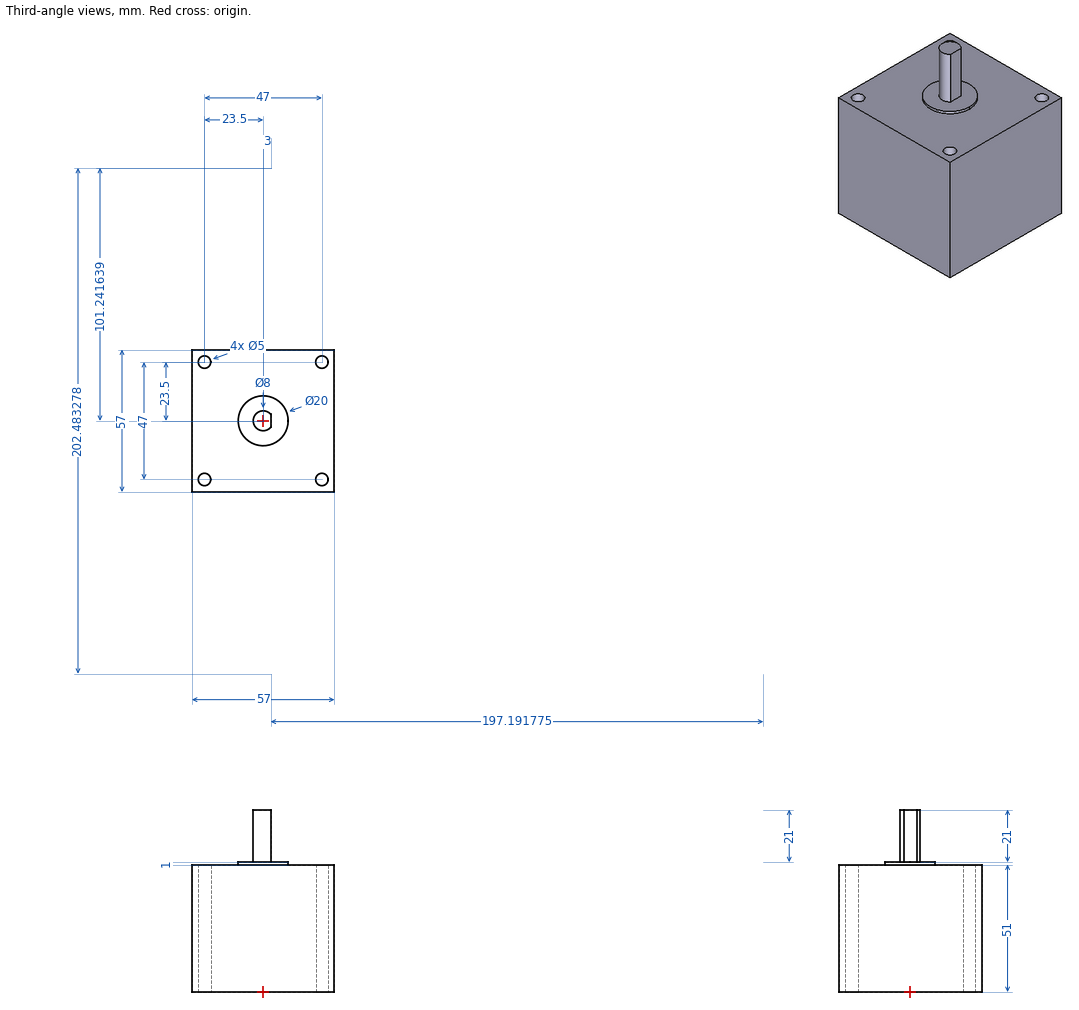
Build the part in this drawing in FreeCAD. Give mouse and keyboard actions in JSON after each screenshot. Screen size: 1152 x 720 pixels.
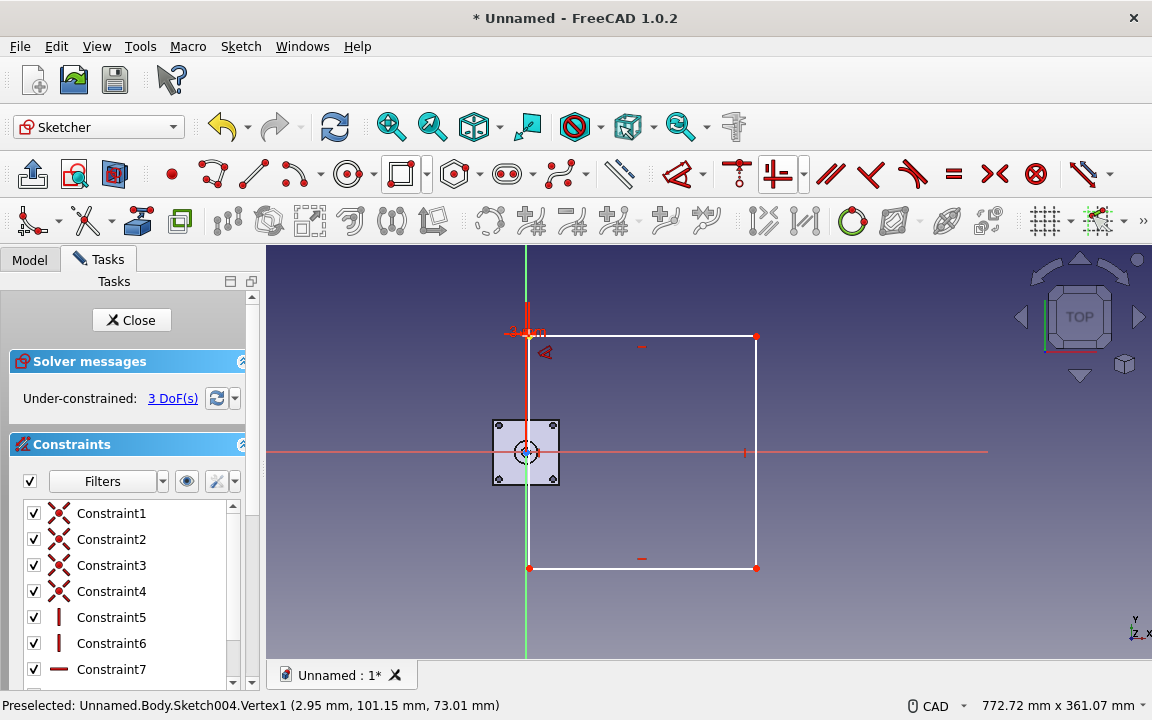
{"action": "scroll", "coordinate": [529, 406], "scroll_direction": "up", "scroll_amount": 7}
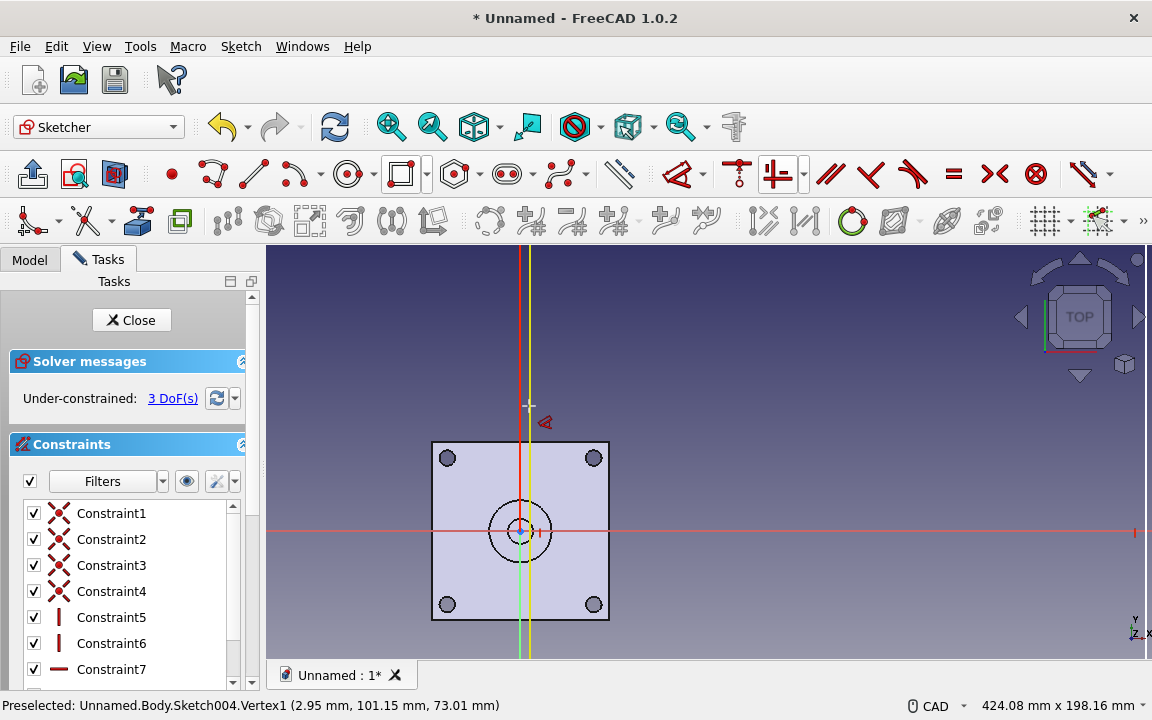
{"action": "left_click", "coordinate": [530, 405]}
{"action": "left_click", "coordinate": [496, 452]}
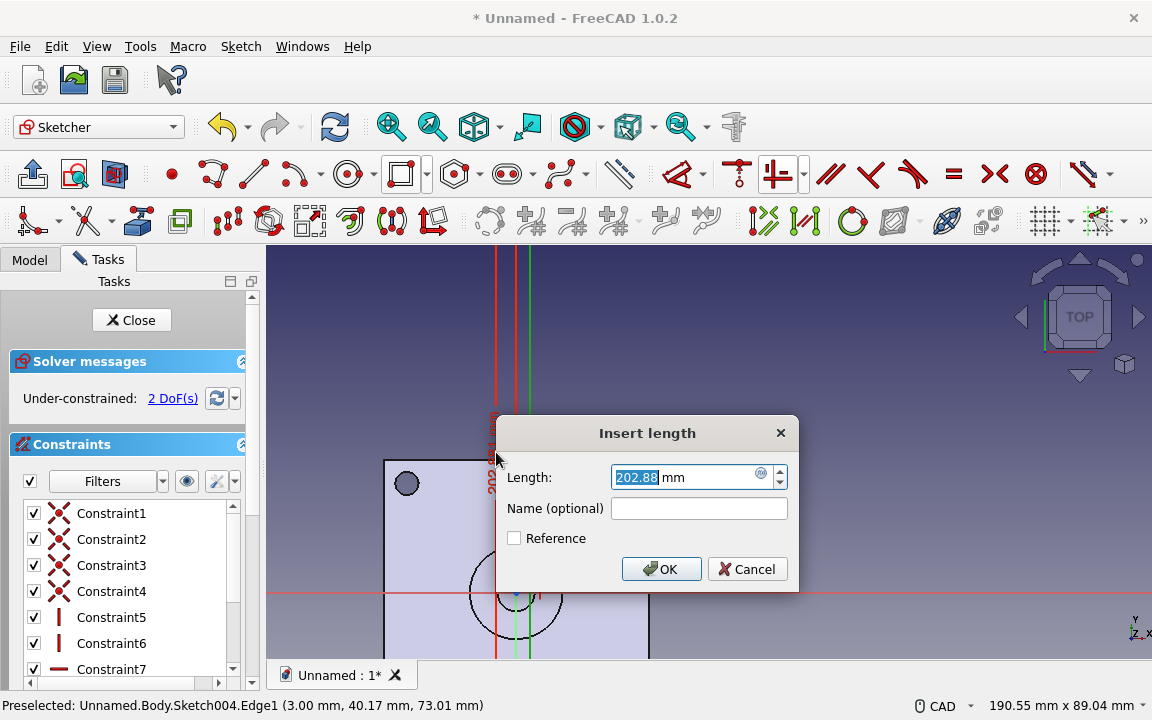
{"action": "type", "text": "202.483278"}
{"action": "key", "text": "Return"}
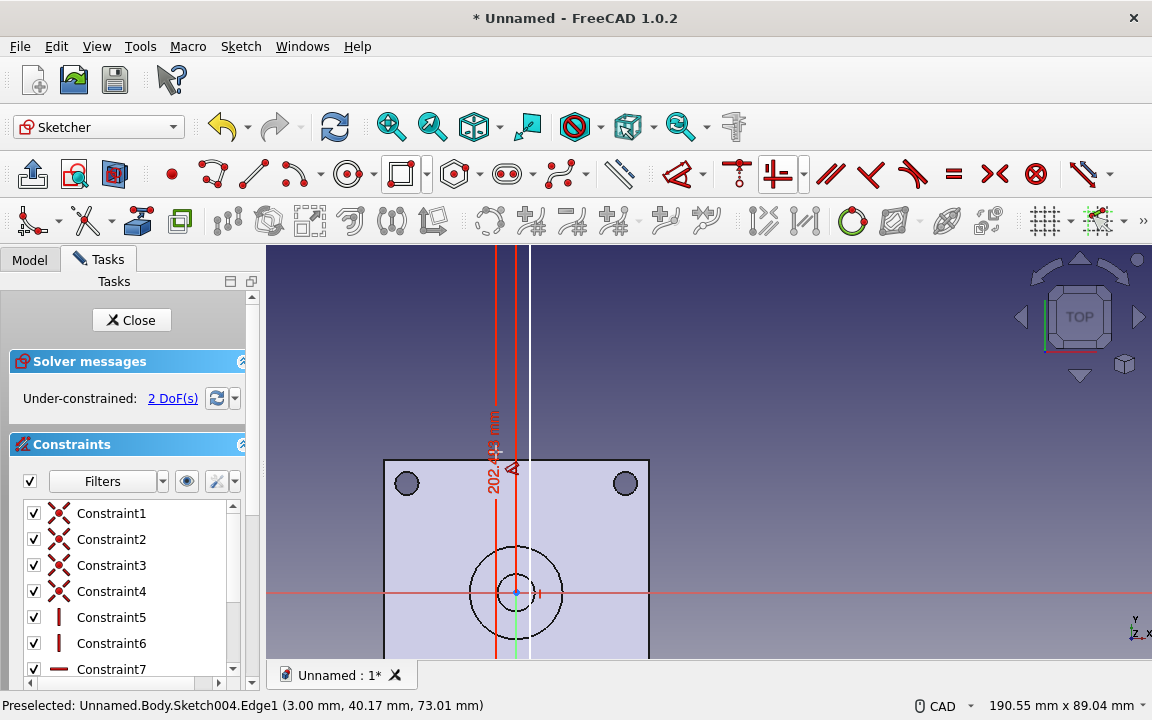
{"action": "scroll", "coordinate": [529, 406], "scroll_direction": "down", "scroll_amount": 7}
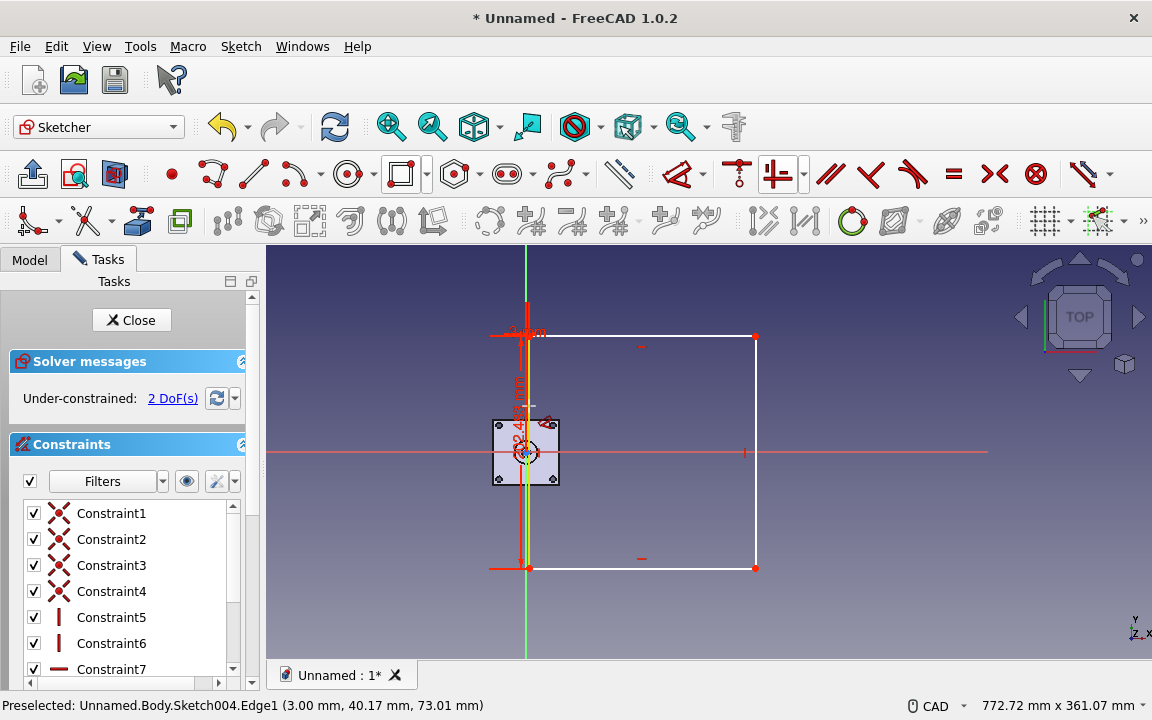
{"action": "left_click", "coordinate": [597, 569]}
{"action": "left_click", "coordinate": [643, 603]}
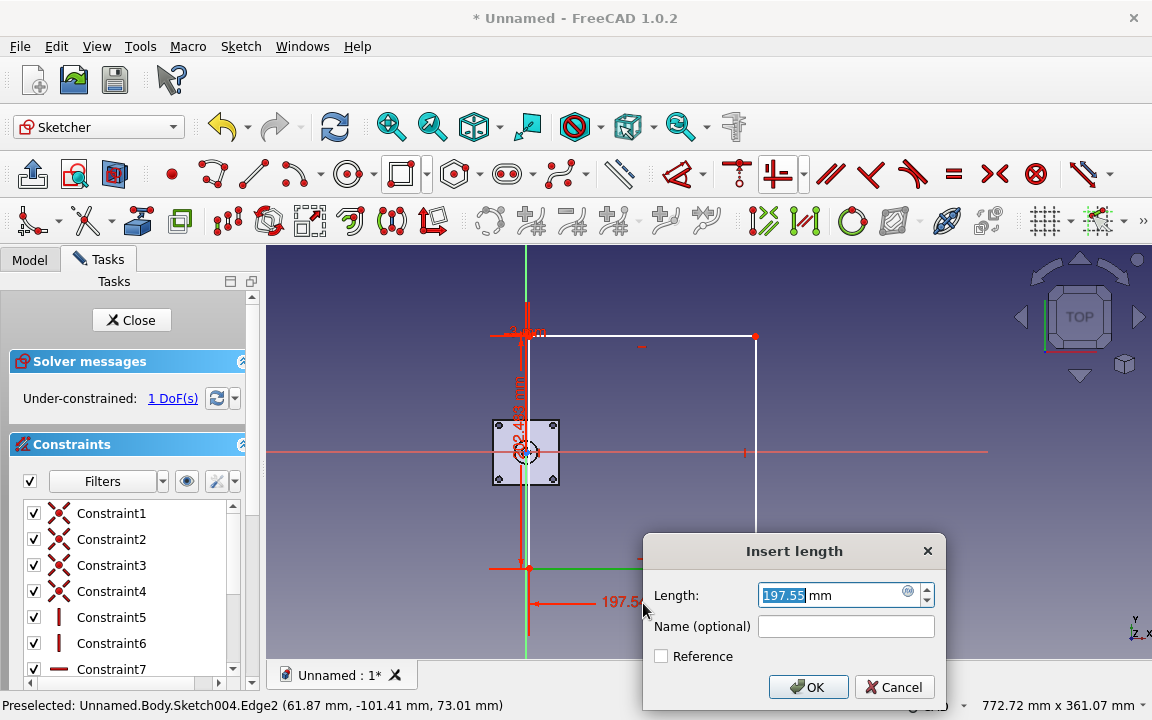
{"action": "type", "text": "197.191775"}
{"action": "key", "text": "Return"}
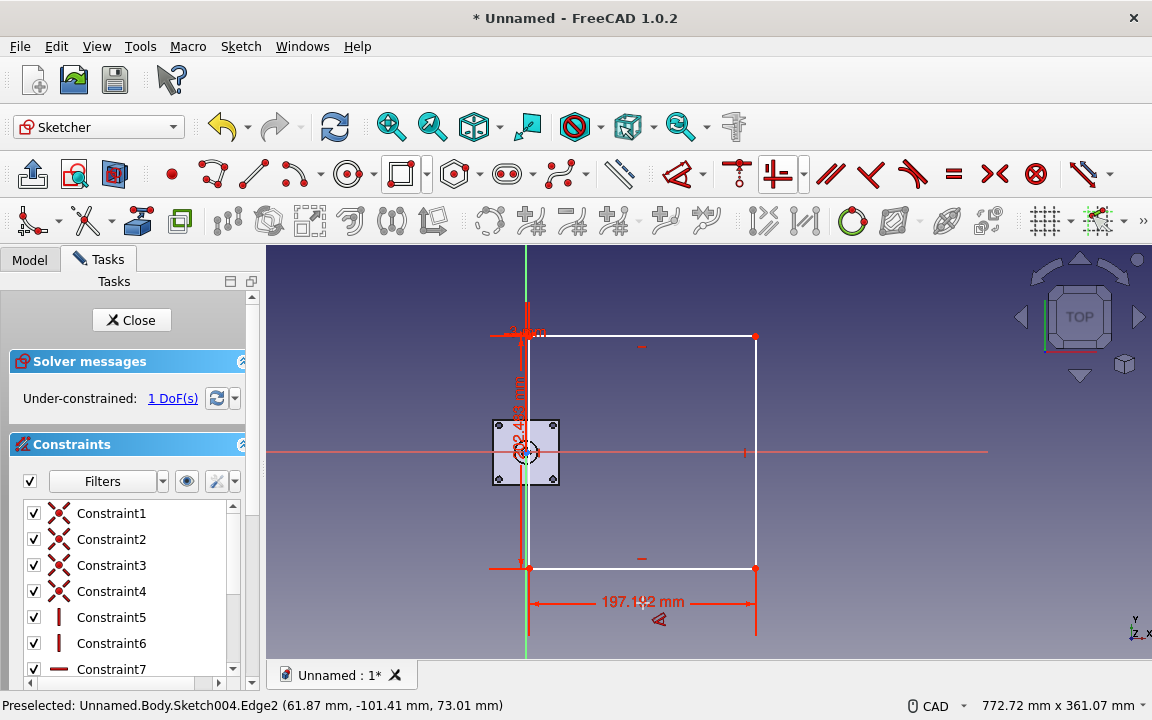
{"action": "left_click", "coordinate": [529, 336]}
{"action": "left_click", "coordinate": [492, 394]}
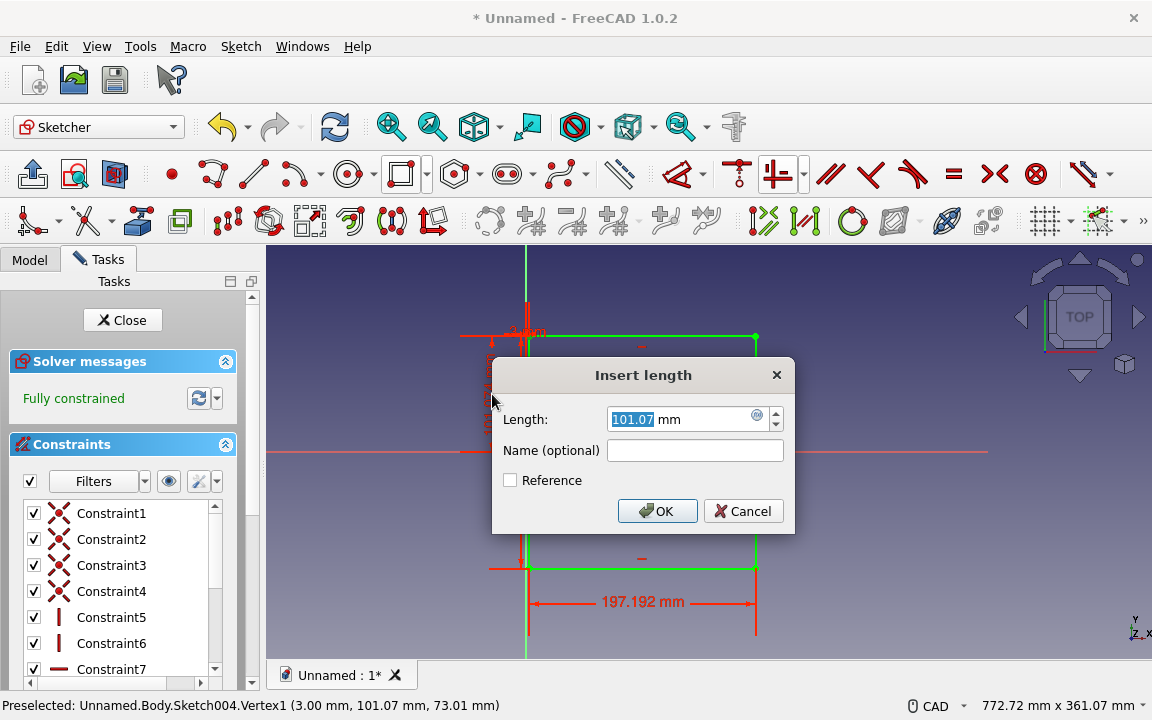
{"action": "type", "text": "101.241639"}
{"action": "key", "text": "Return"}
{"action": "key", "text": "Escape"}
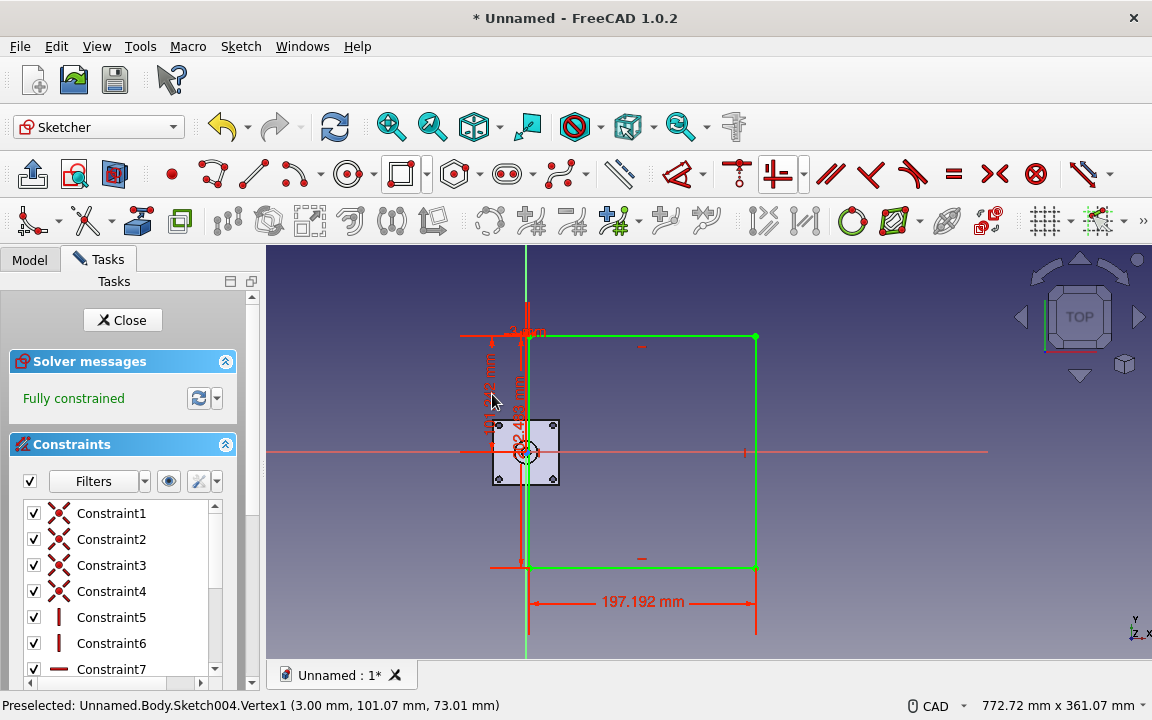
{"action": "left_click", "coordinate": [123, 320]}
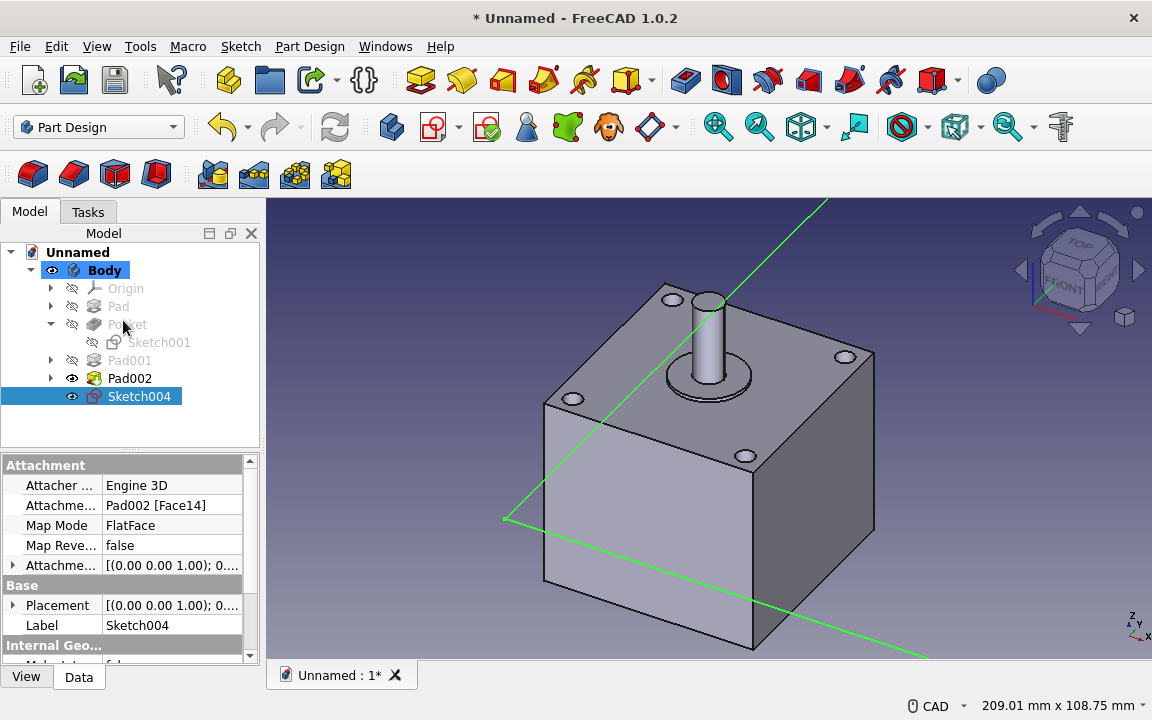
{"action": "left_click", "coordinate": [686, 80]}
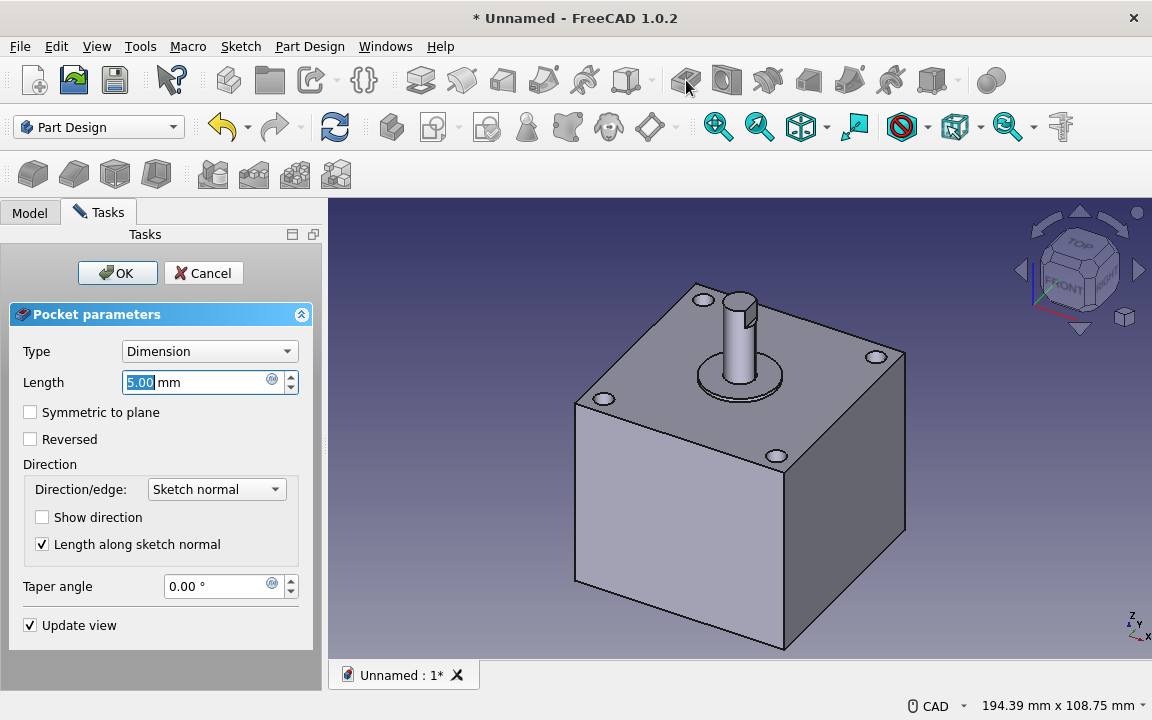
{"action": "type", "text": "21"}
{"action": "key", "text": "Tab"}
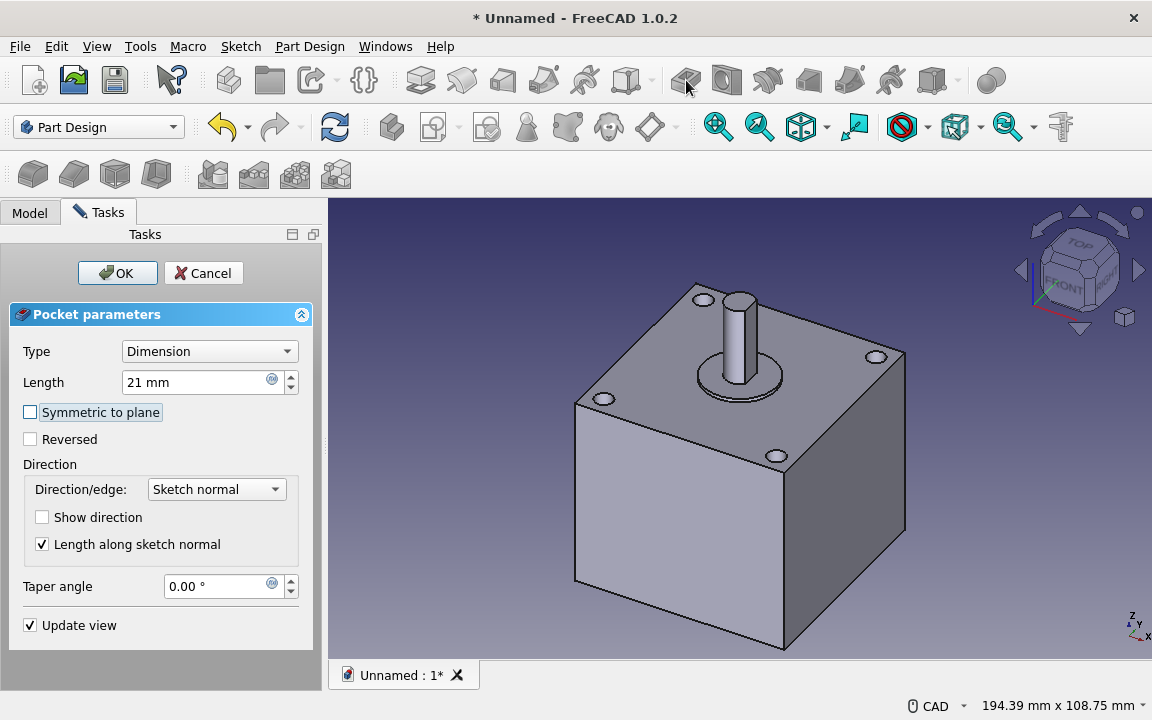
{"action": "left_click", "coordinate": [118, 273]}